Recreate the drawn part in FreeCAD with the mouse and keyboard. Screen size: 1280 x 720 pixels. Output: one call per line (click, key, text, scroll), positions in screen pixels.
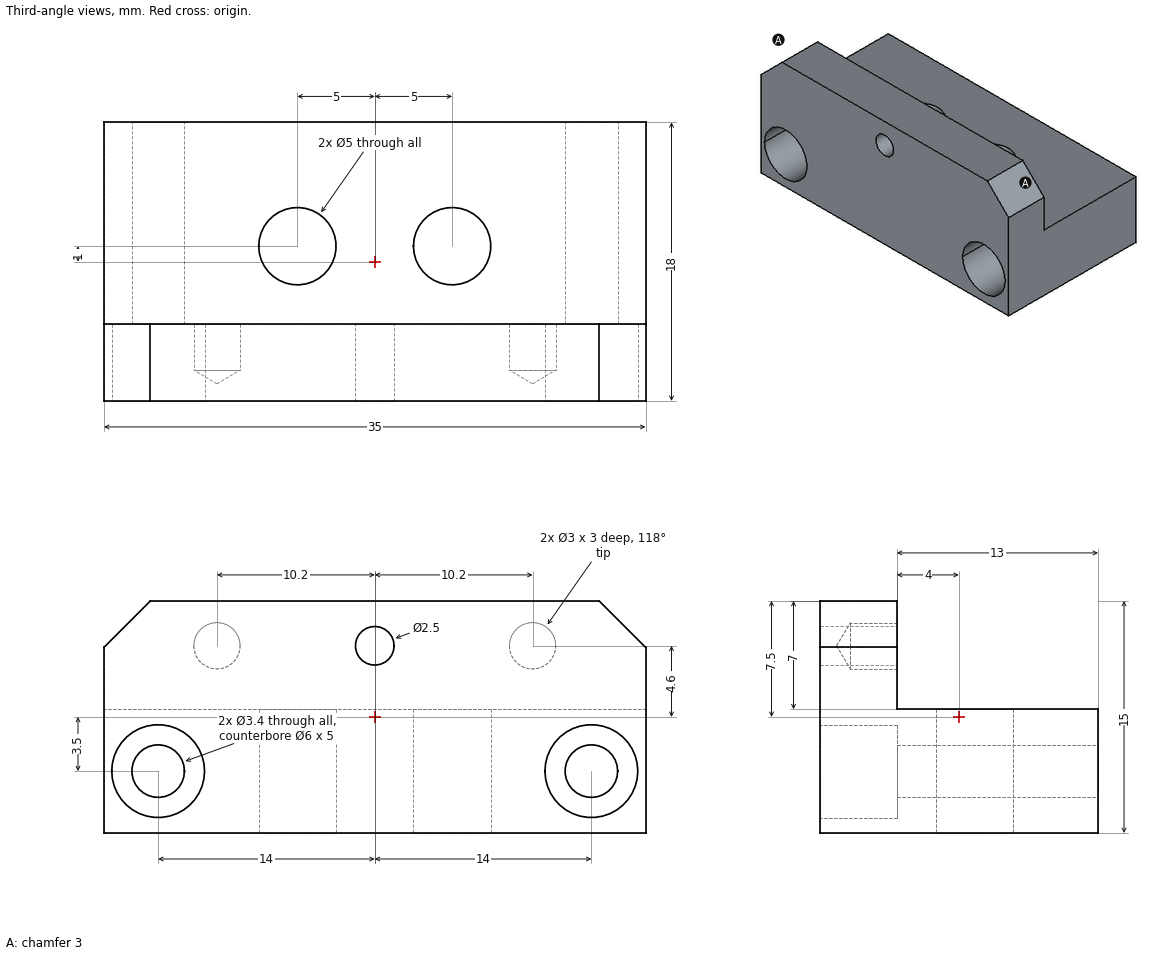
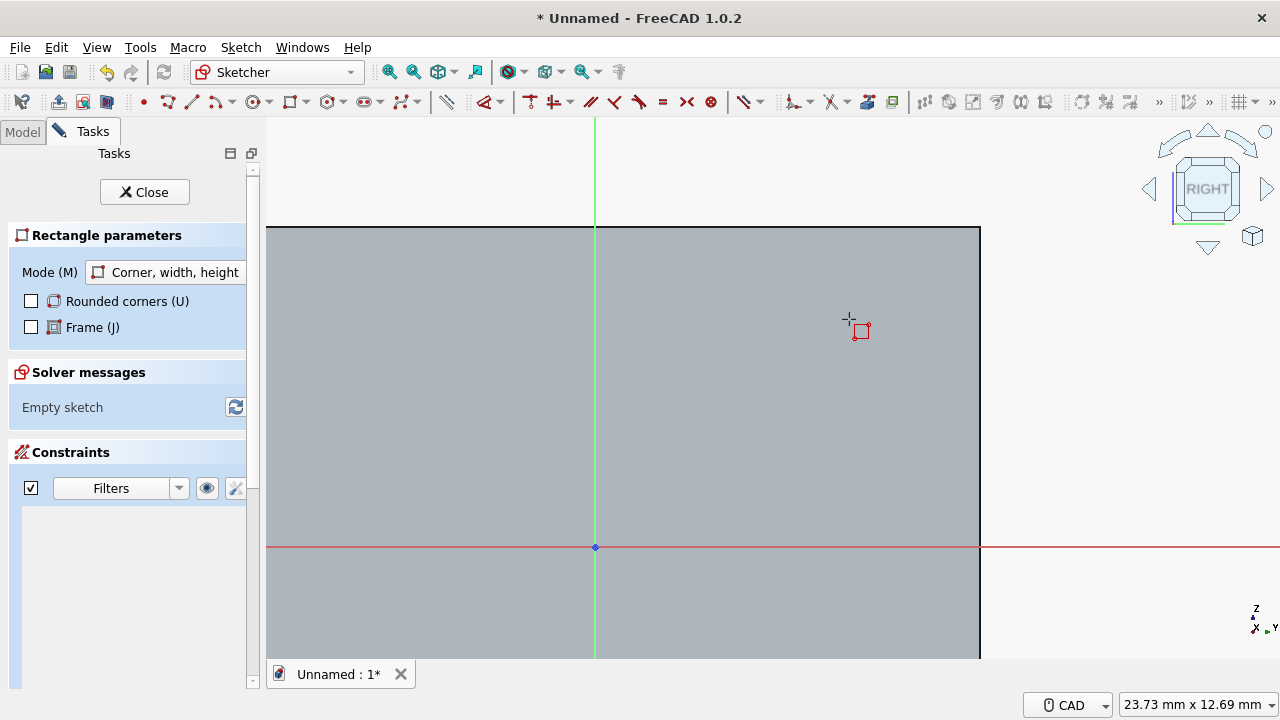
click(424, 227)
click(980, 526)
key(Escape)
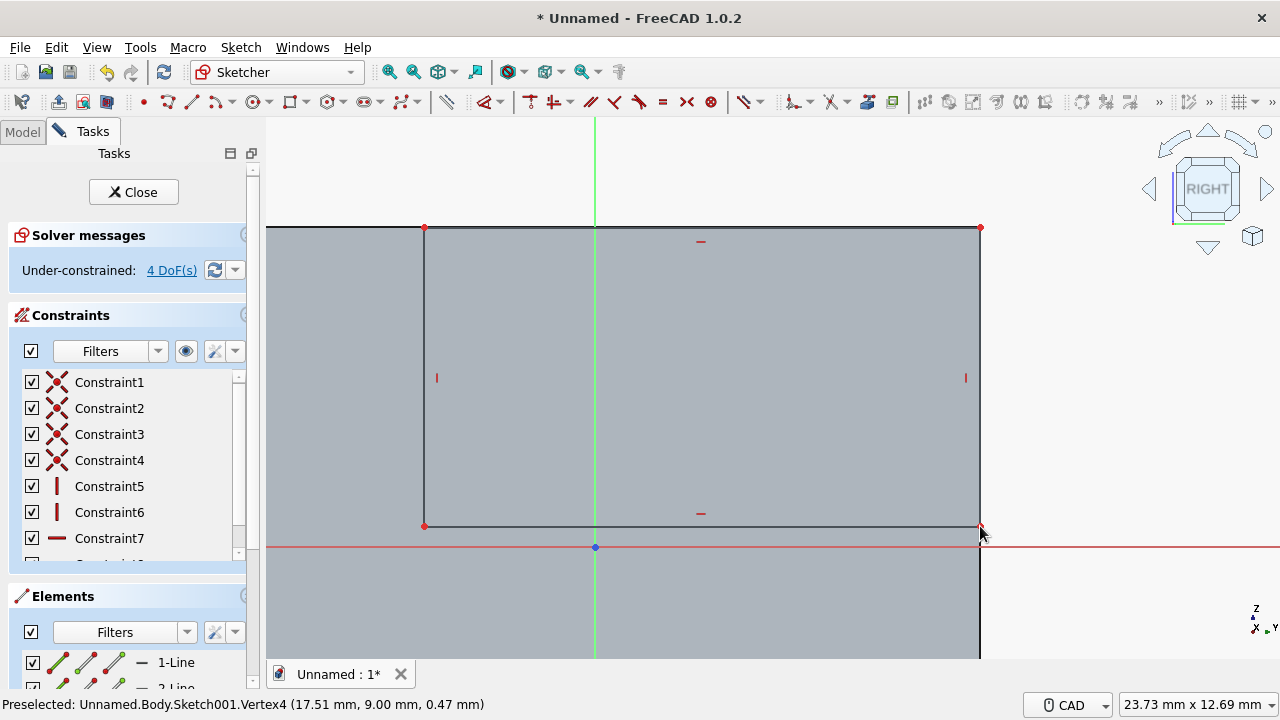
key(d)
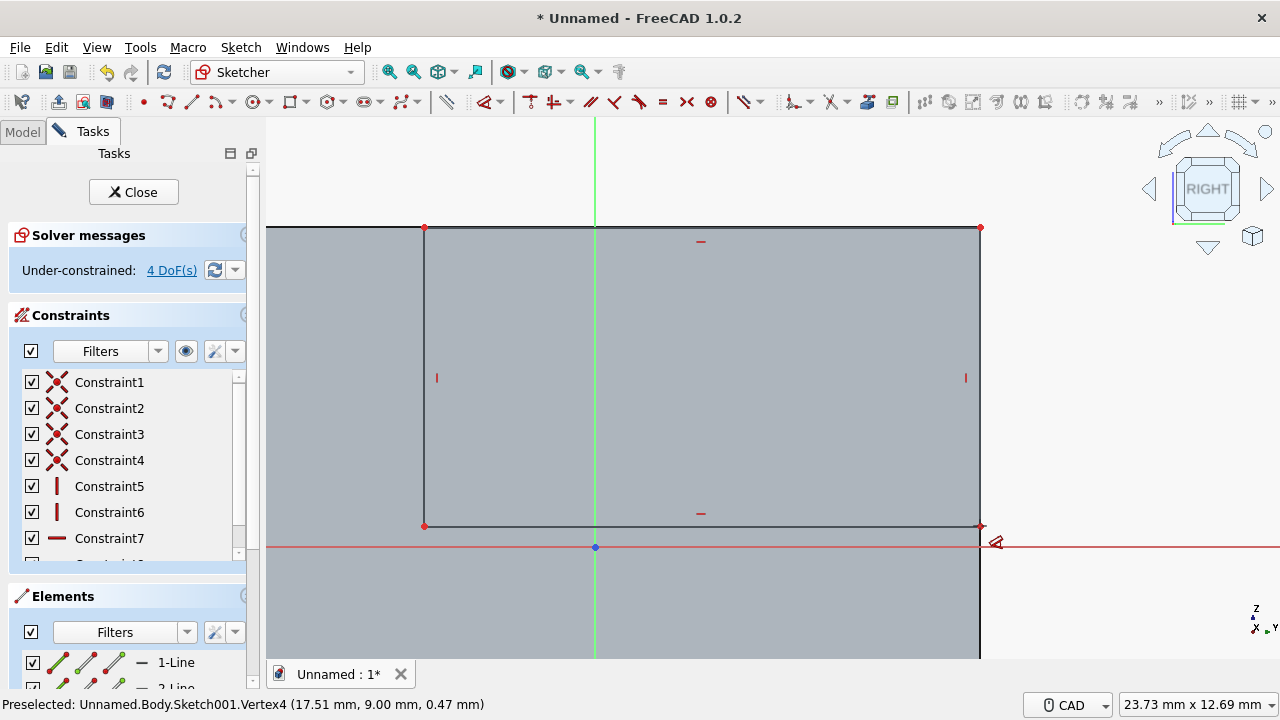
click(424, 318)
click(390, 377)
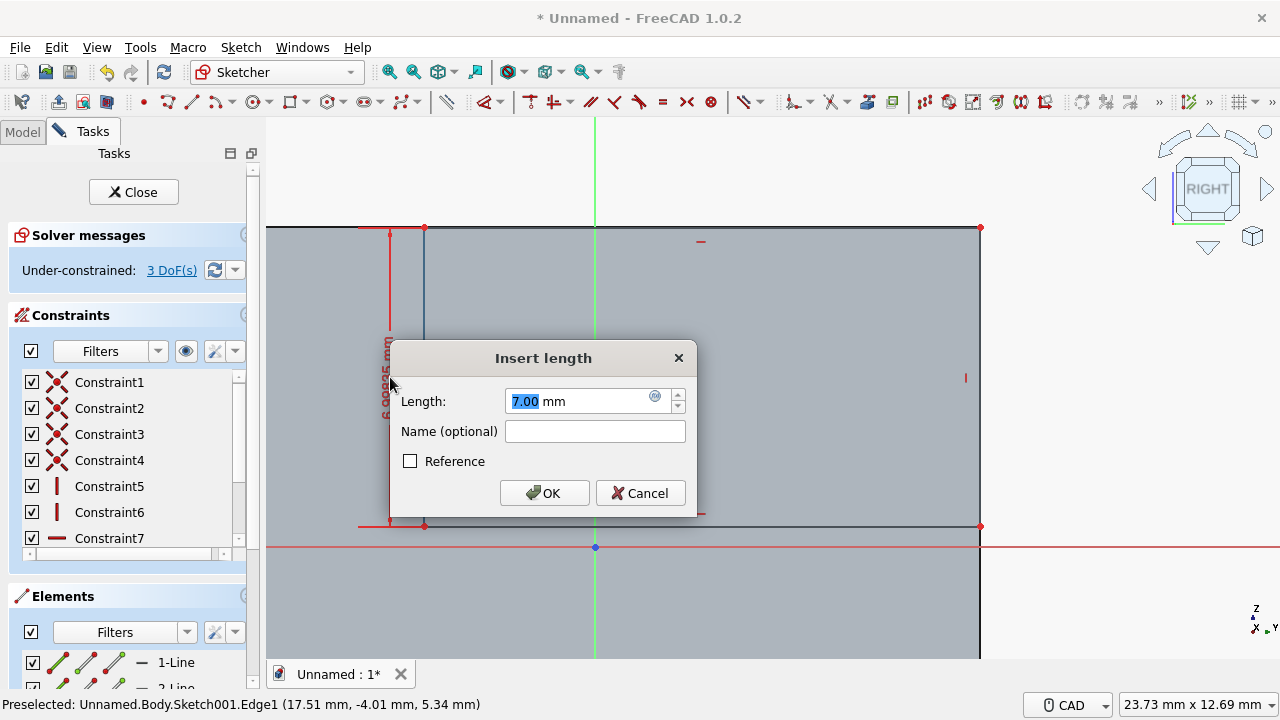
text(7)
key(Return)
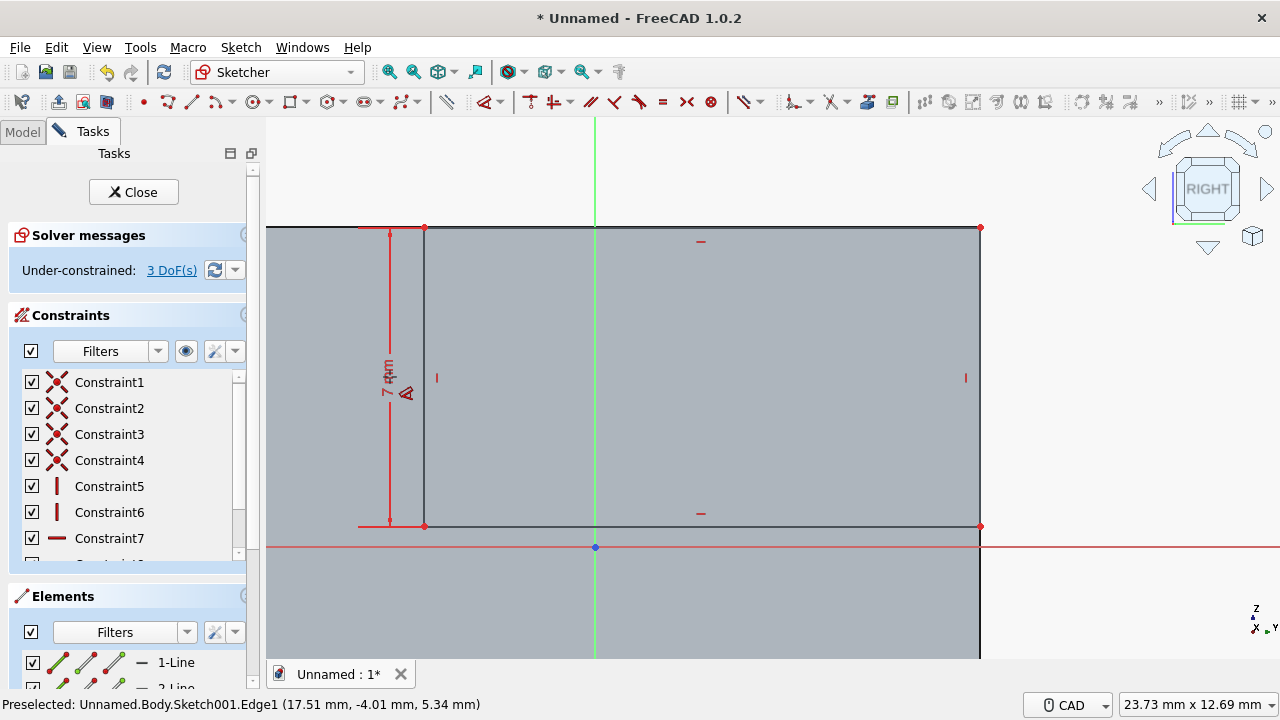
click(813, 527)
click(702, 561)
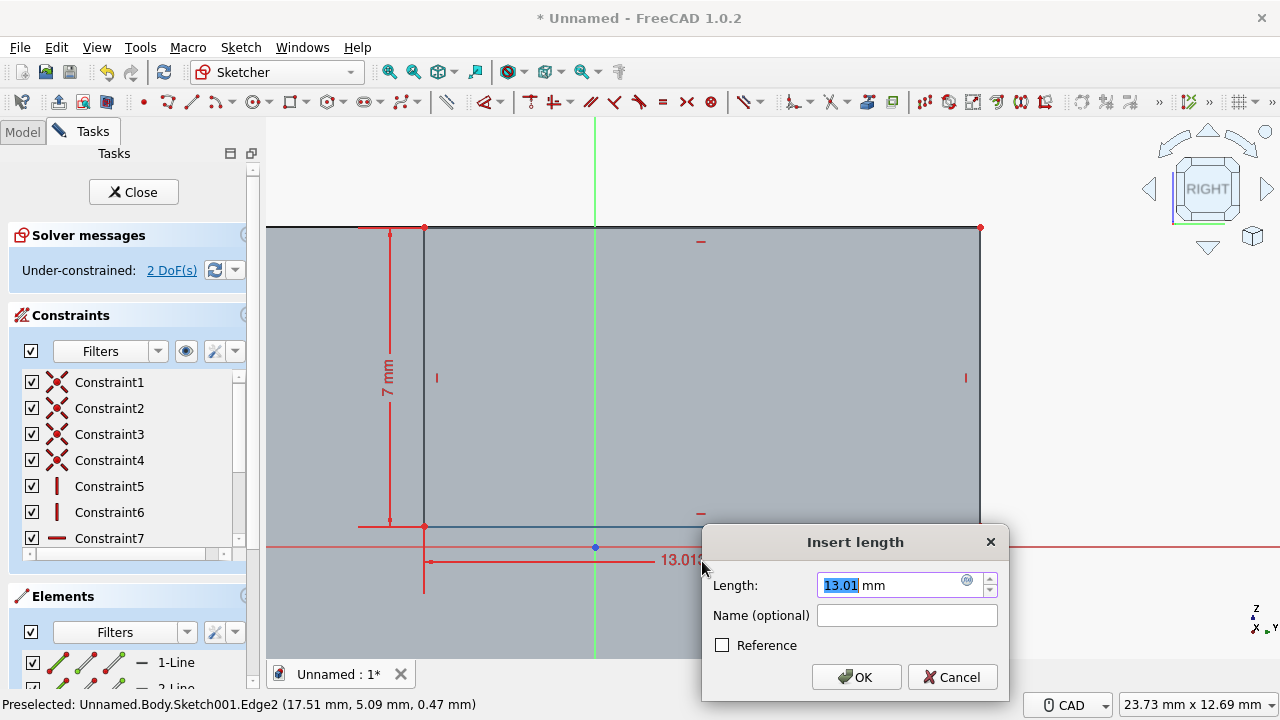
text(13)
key(Return)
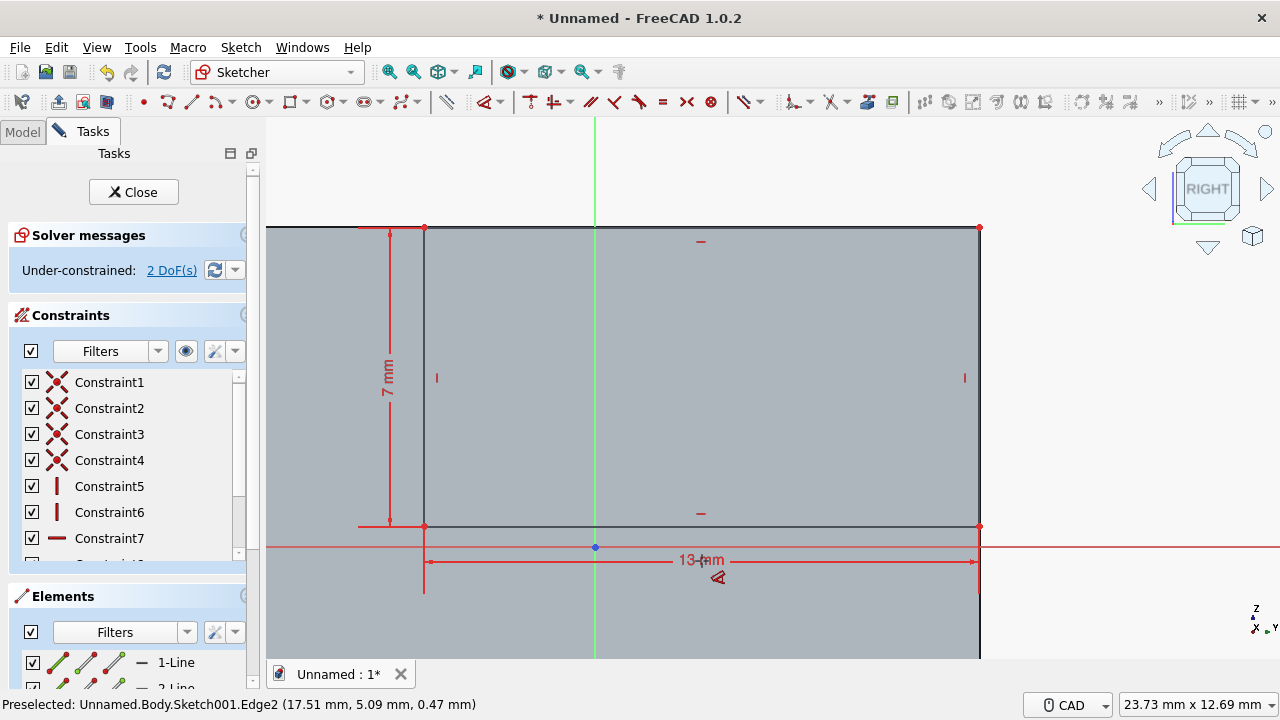
click(424, 228)
click(510, 581)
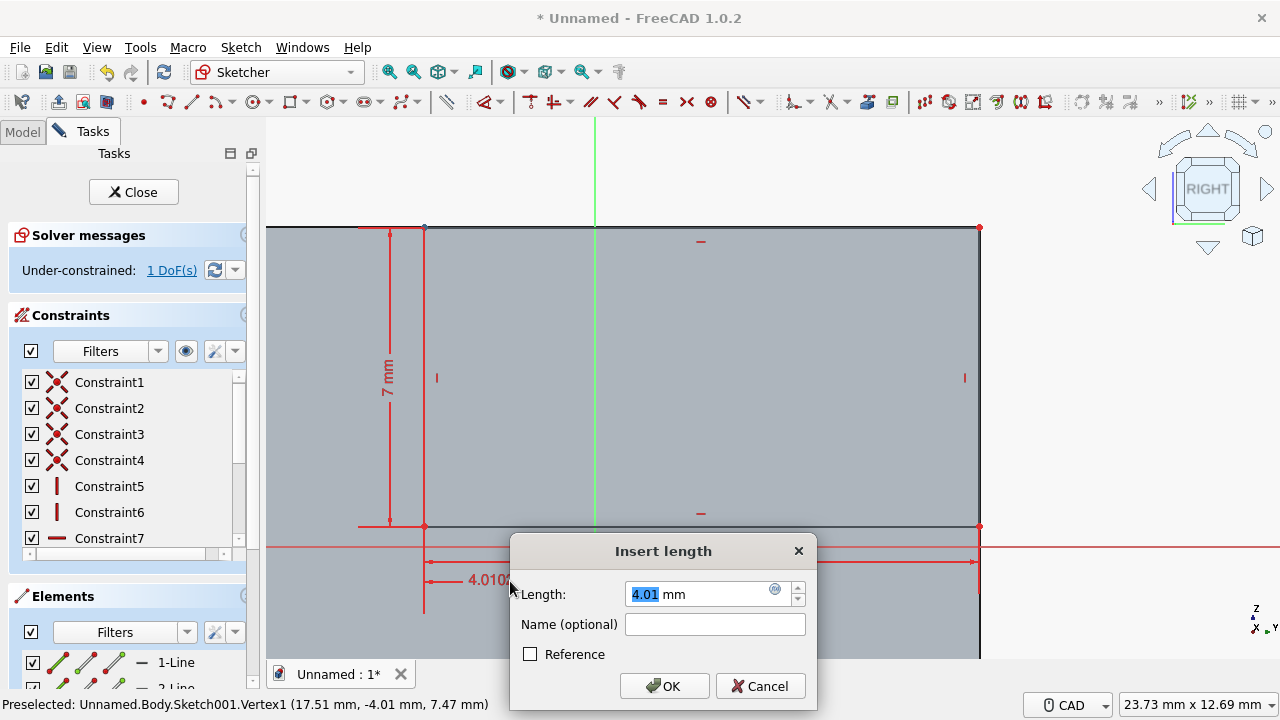
text(4)
key(Return)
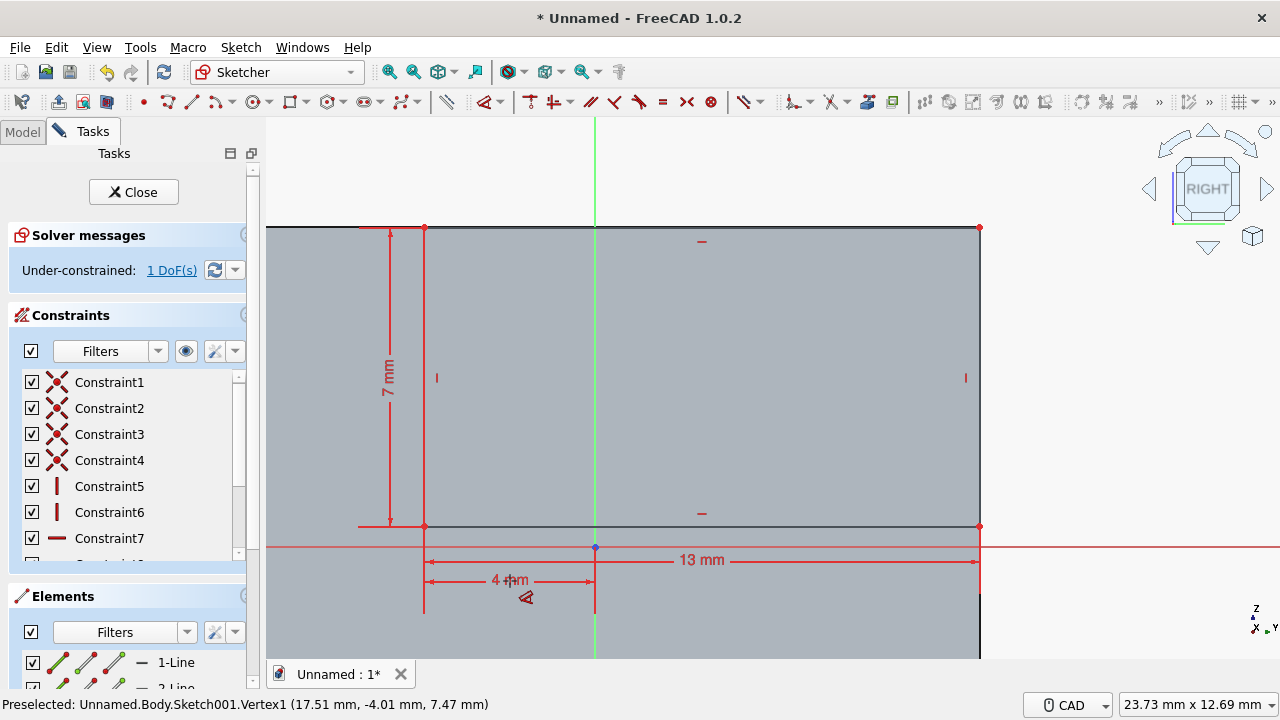
click(424, 228)
click(390, 314)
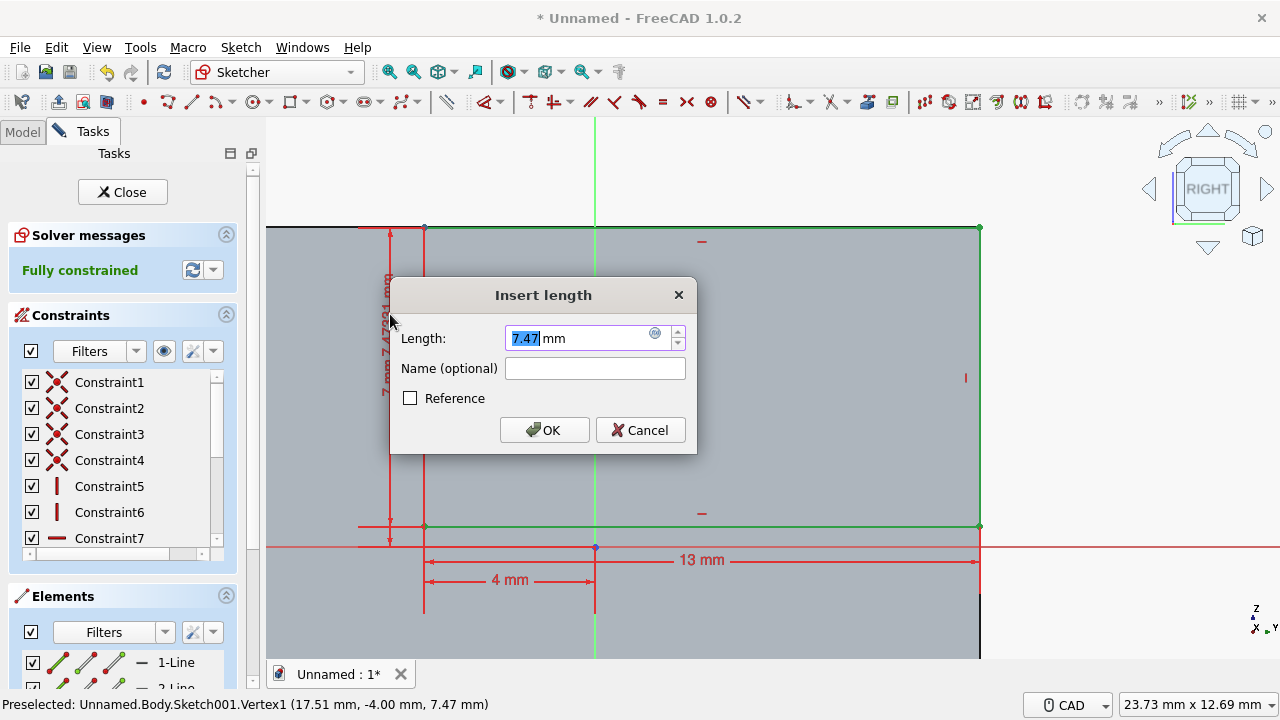
text(7.5)
key(Return)
key(Escape)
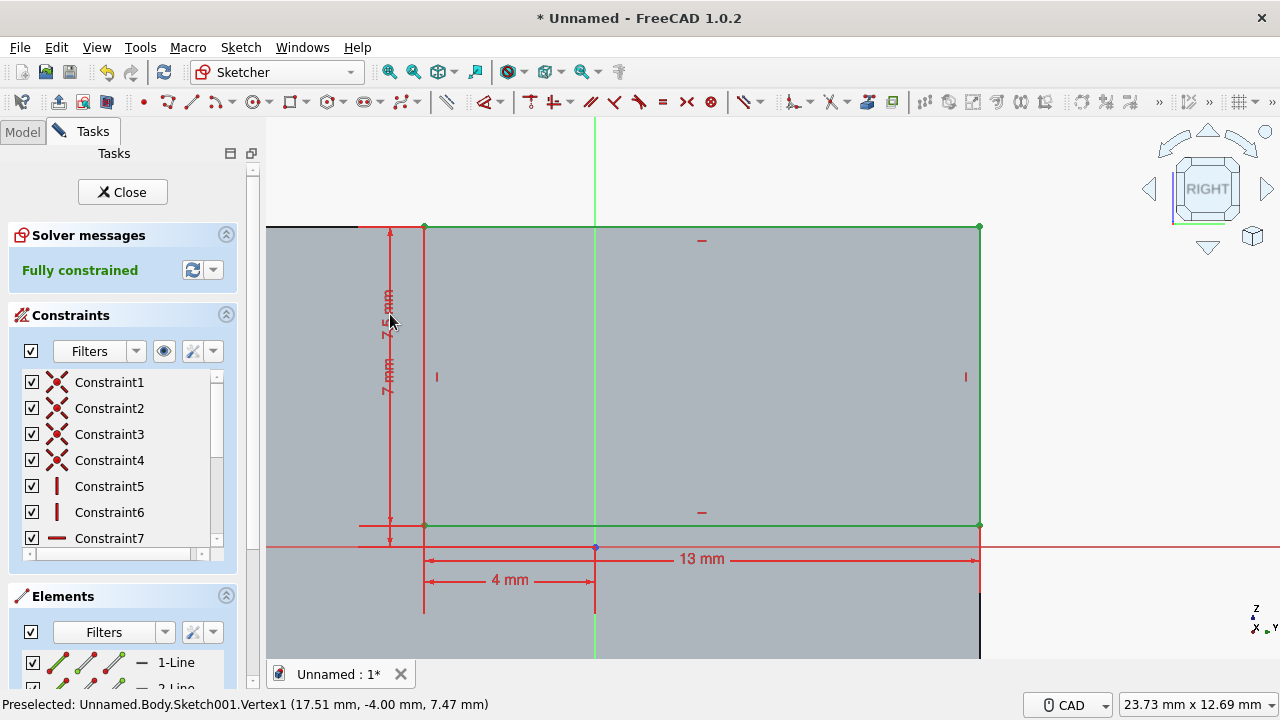
click(123, 192)